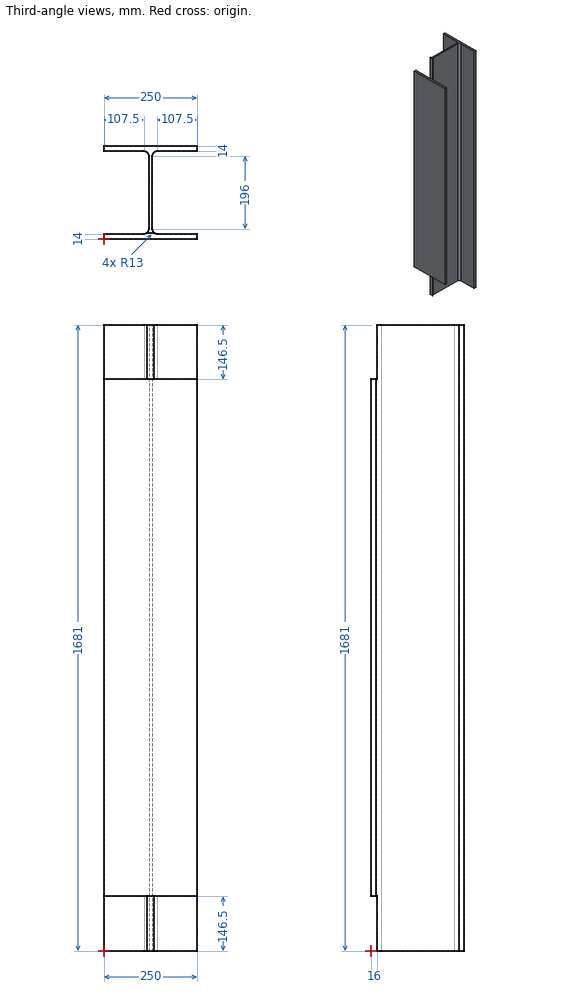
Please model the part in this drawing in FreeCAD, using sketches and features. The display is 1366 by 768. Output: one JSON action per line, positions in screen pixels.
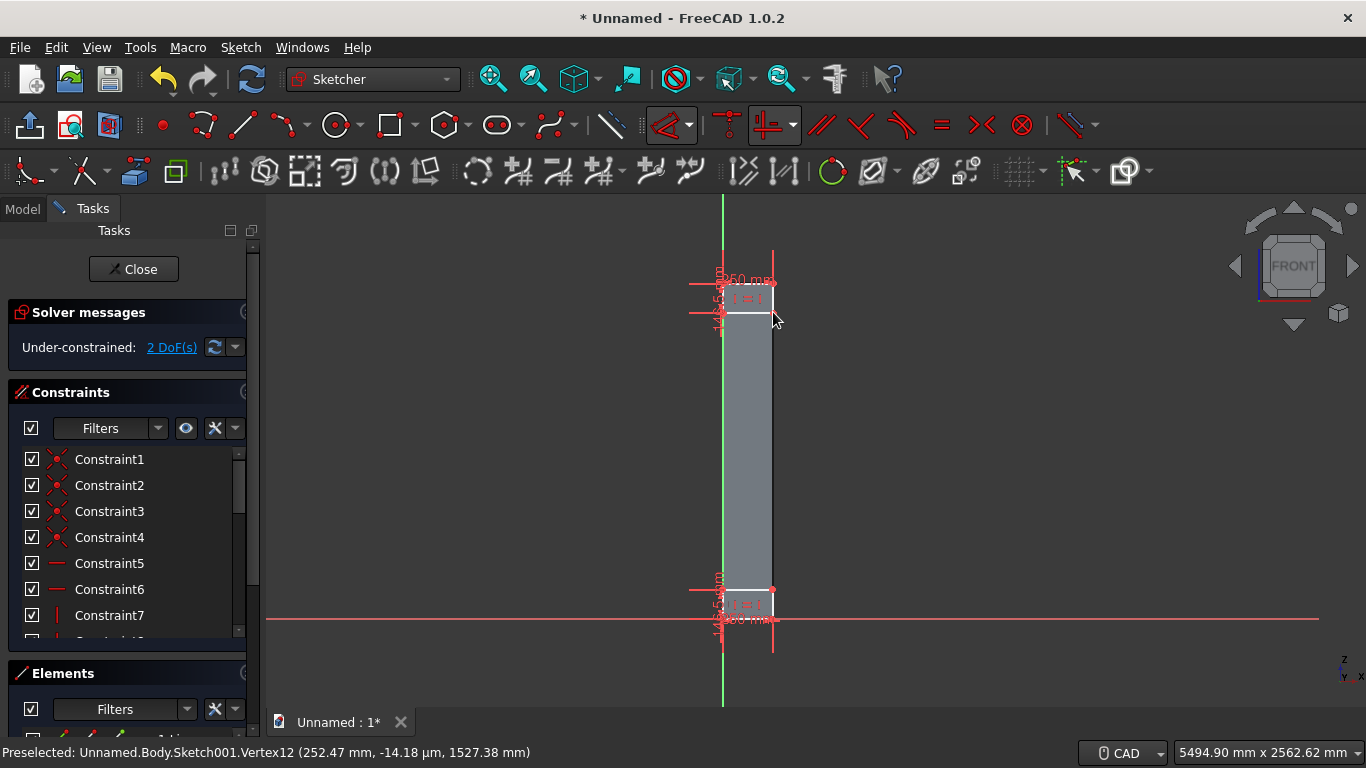
{"action": "left_click", "coordinate": [723, 284]}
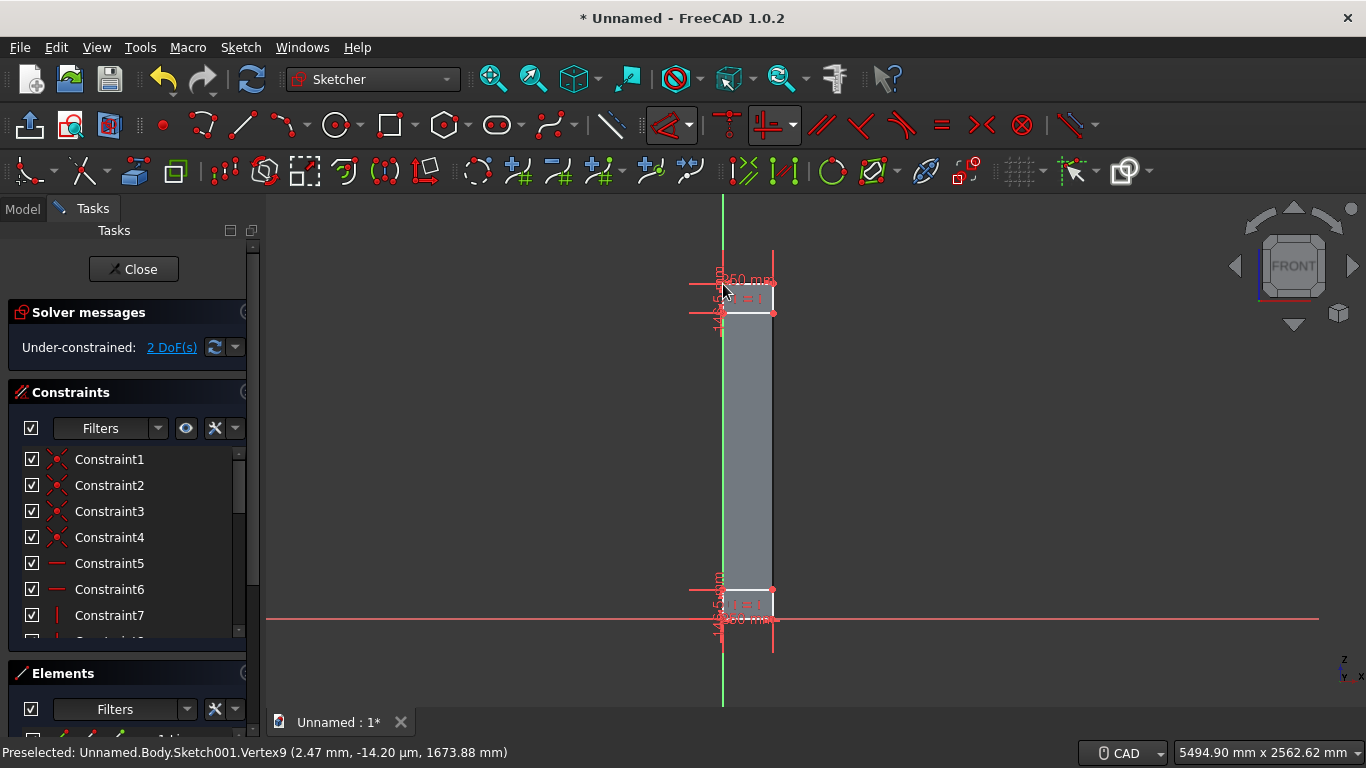
{"action": "left_click", "coordinate": [723, 548]}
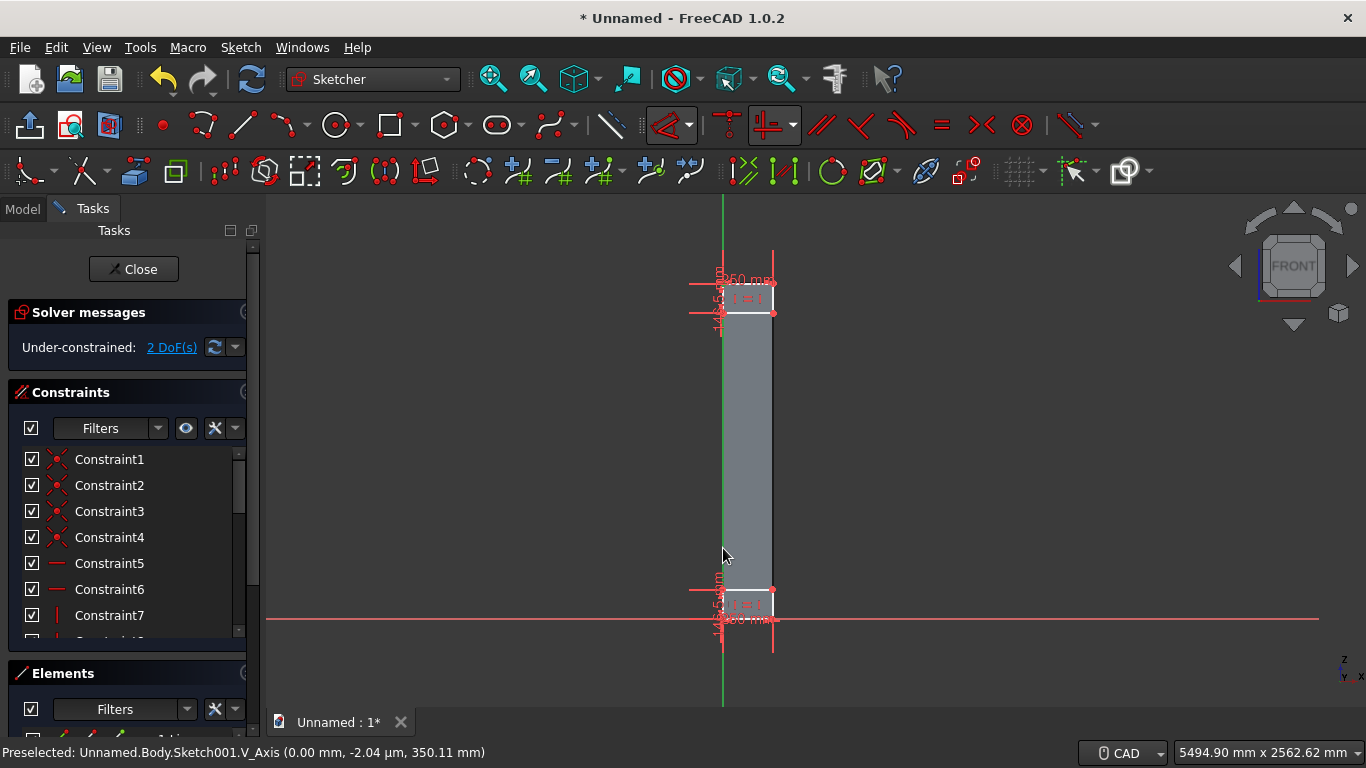
{"action": "left_click", "coordinate": [728, 126]}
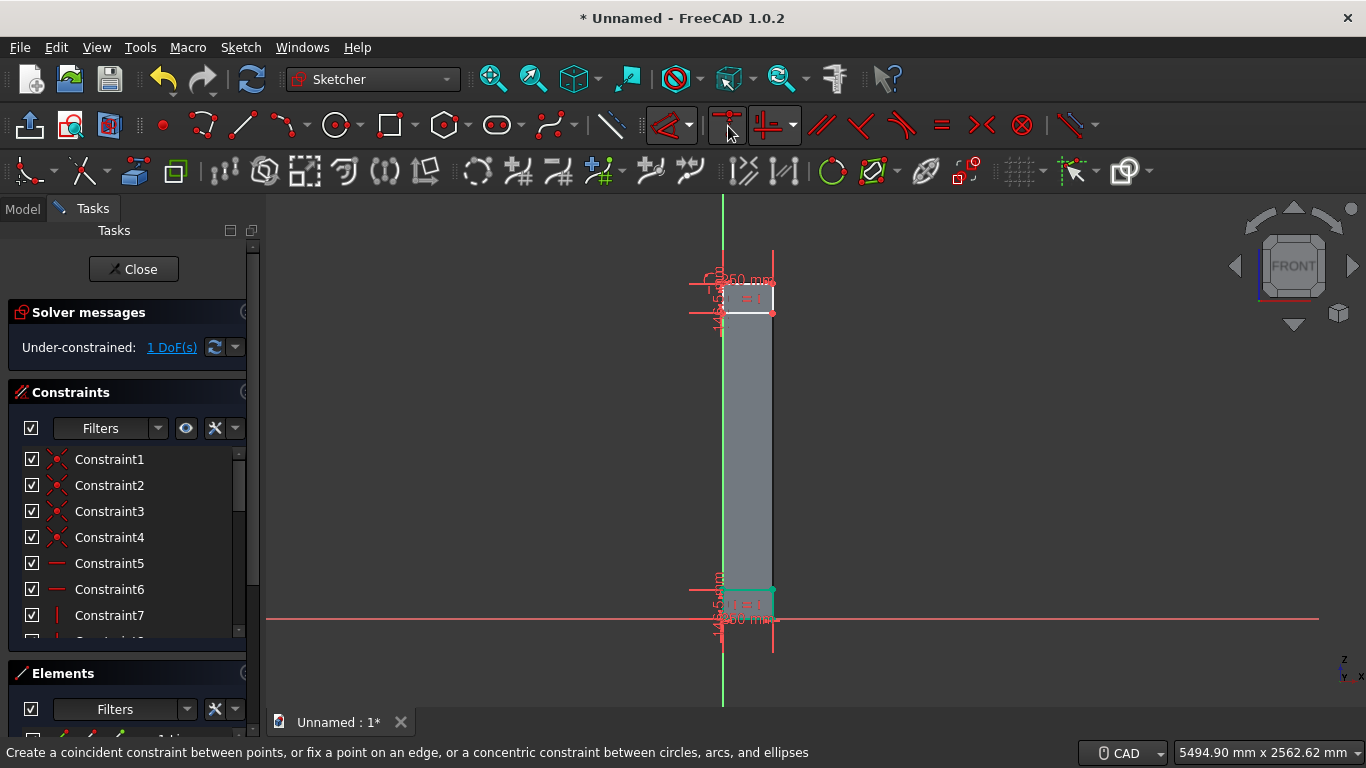
{"action": "left_click", "coordinate": [723, 284]}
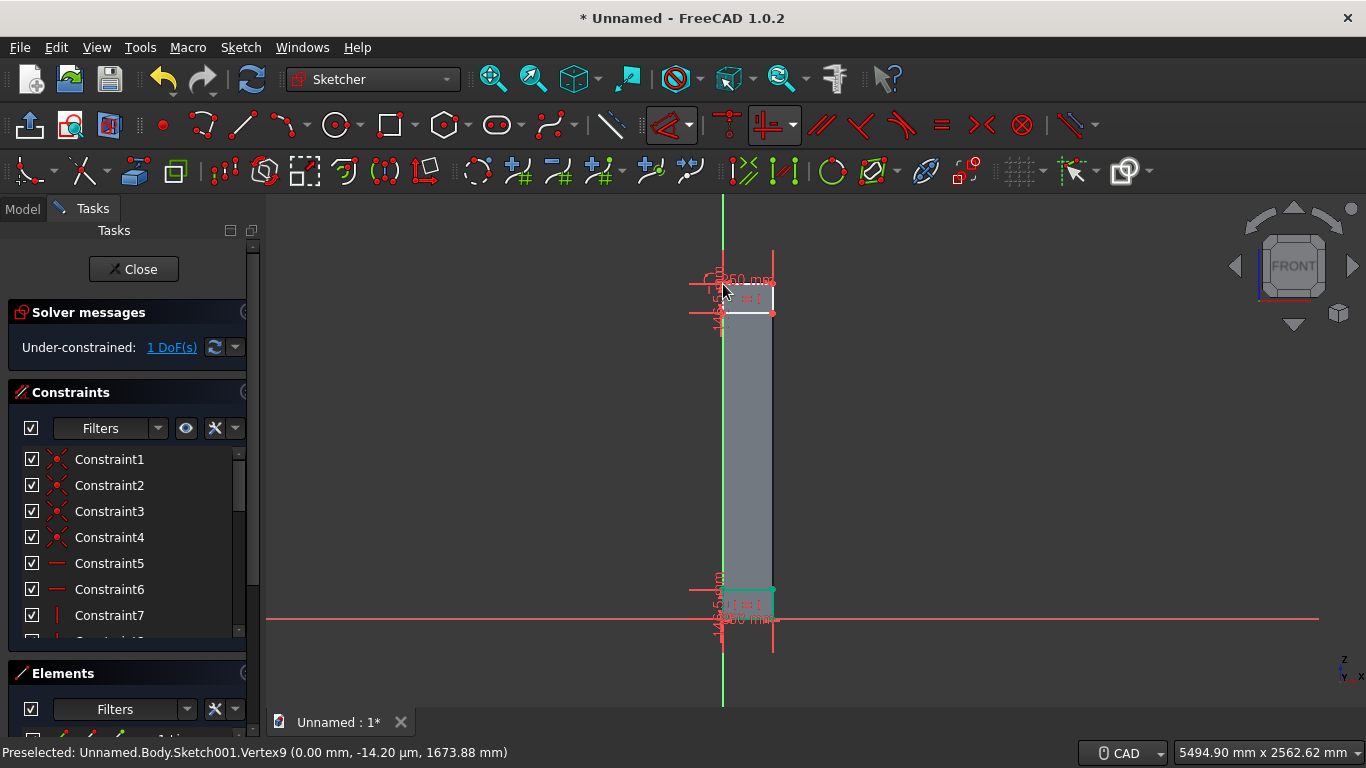
{"action": "key", "text": "i"}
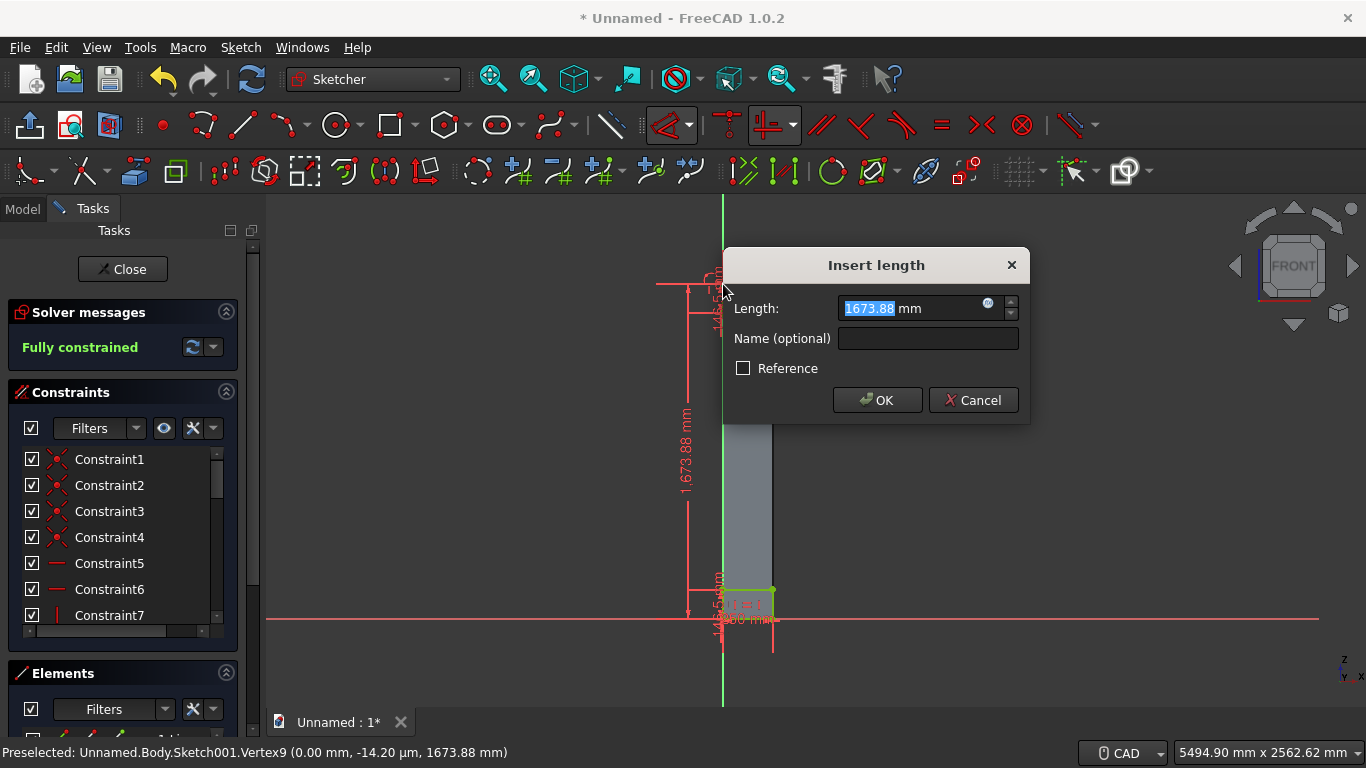
{"action": "type", "text": "1681"}
{"action": "key", "text": "Return"}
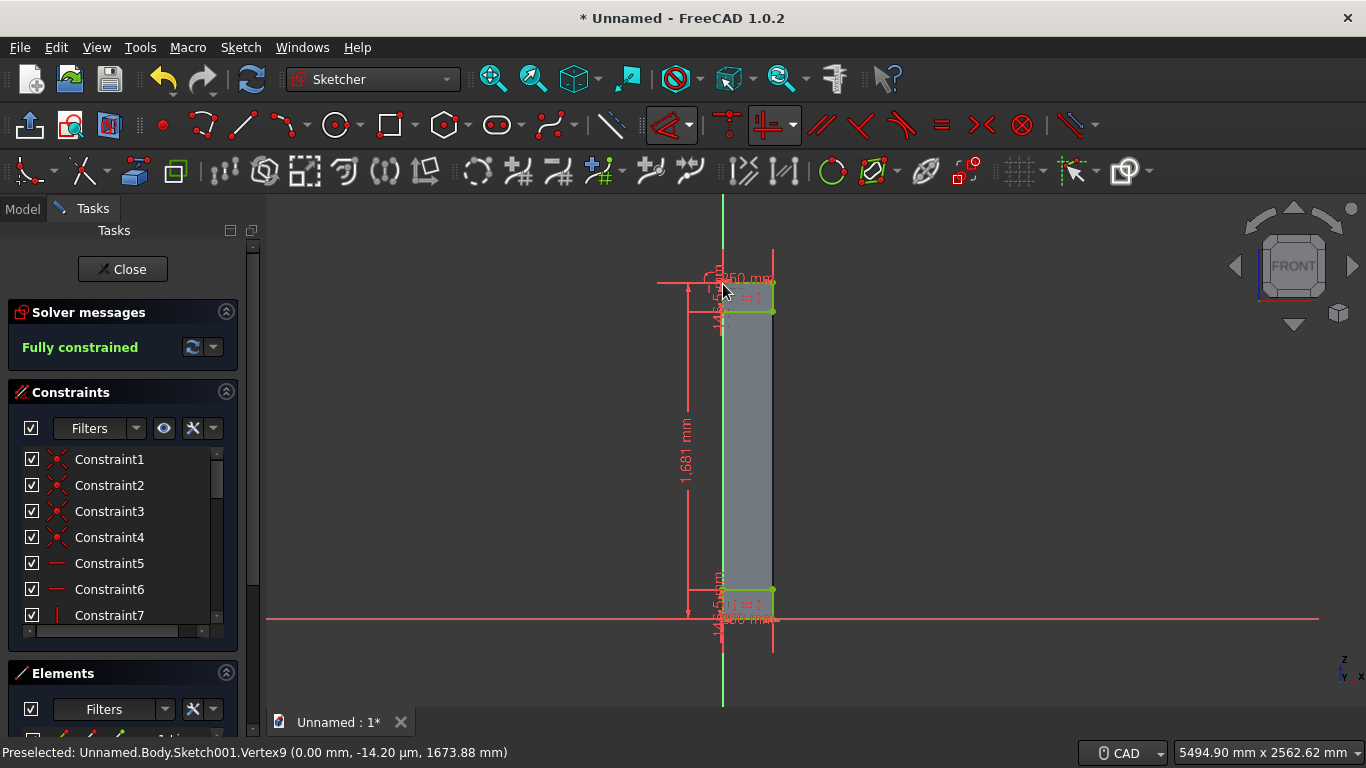
{"action": "left_click", "coordinate": [123, 269]}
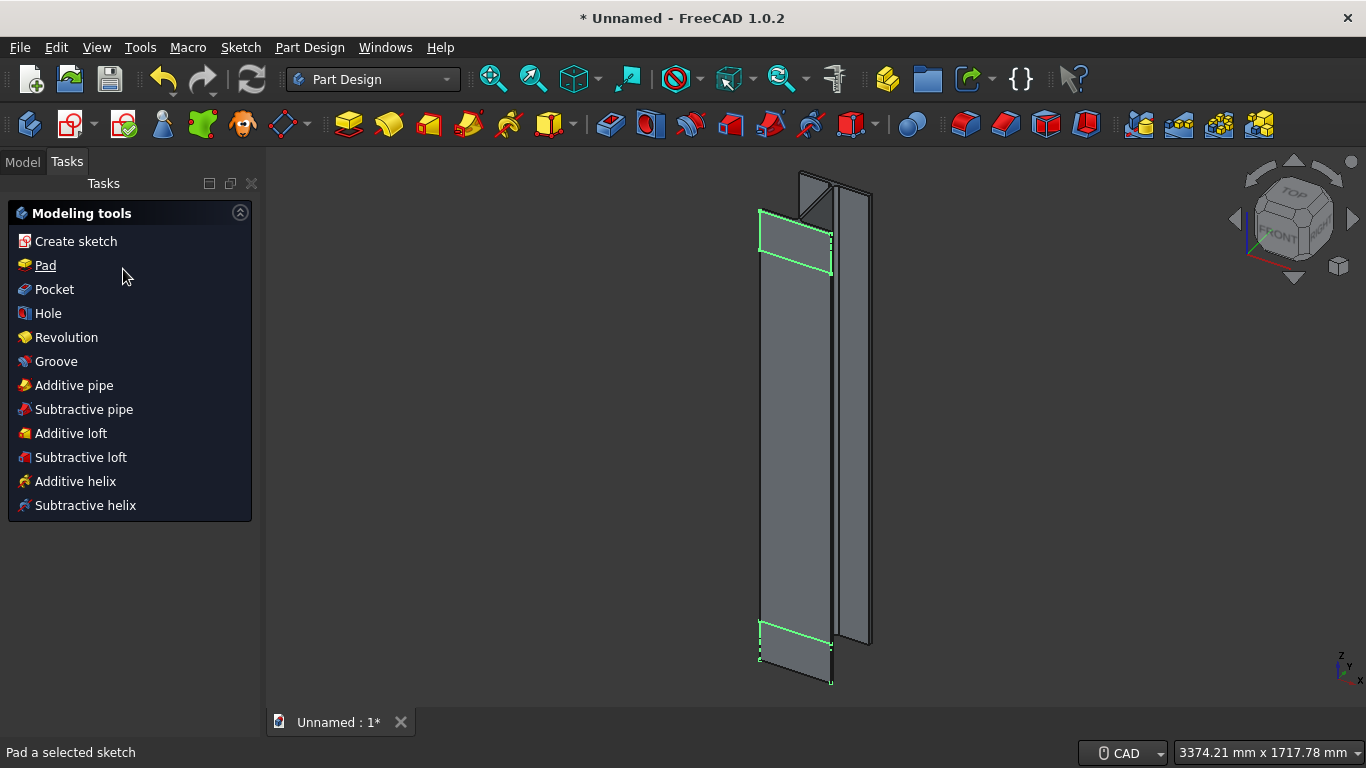
{"action": "left_click", "coordinate": [612, 124]}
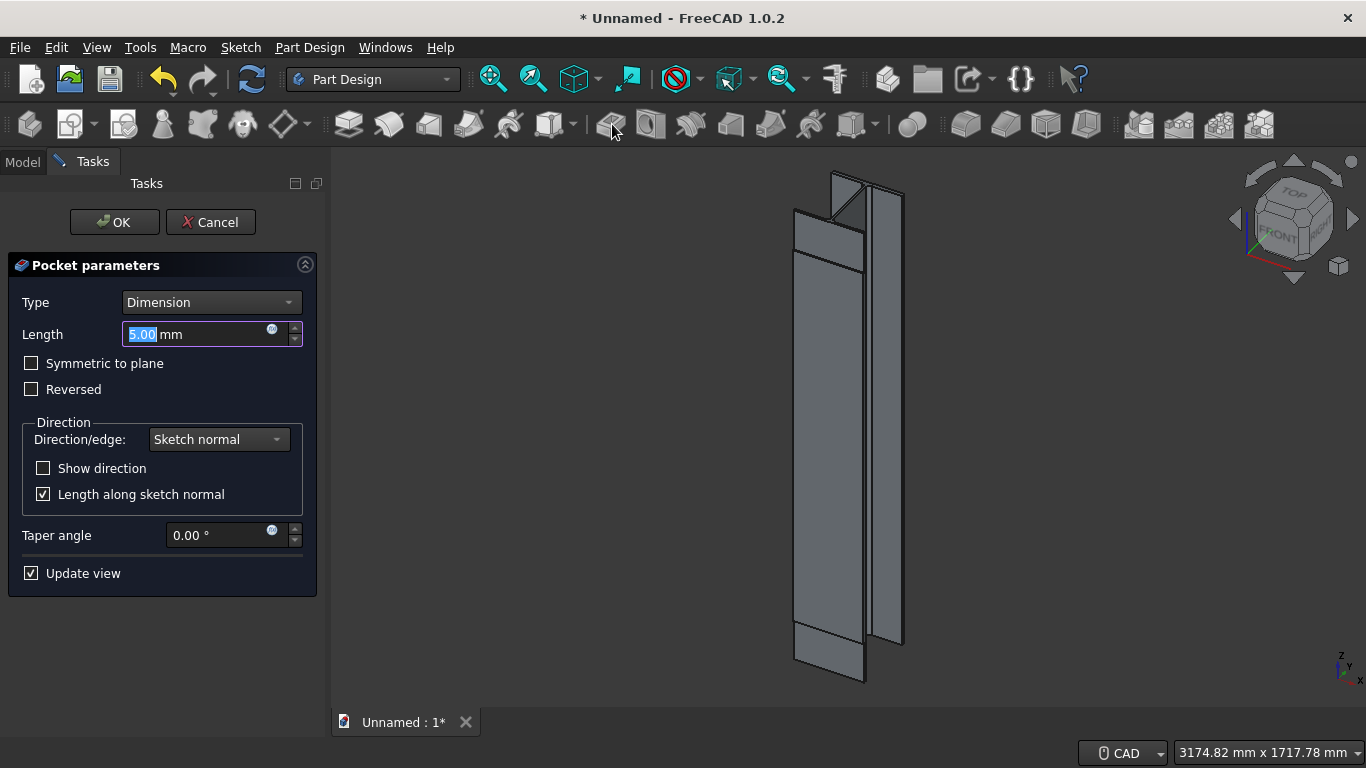
{"action": "type", "text": "16"}
{"action": "key", "text": "Tab"}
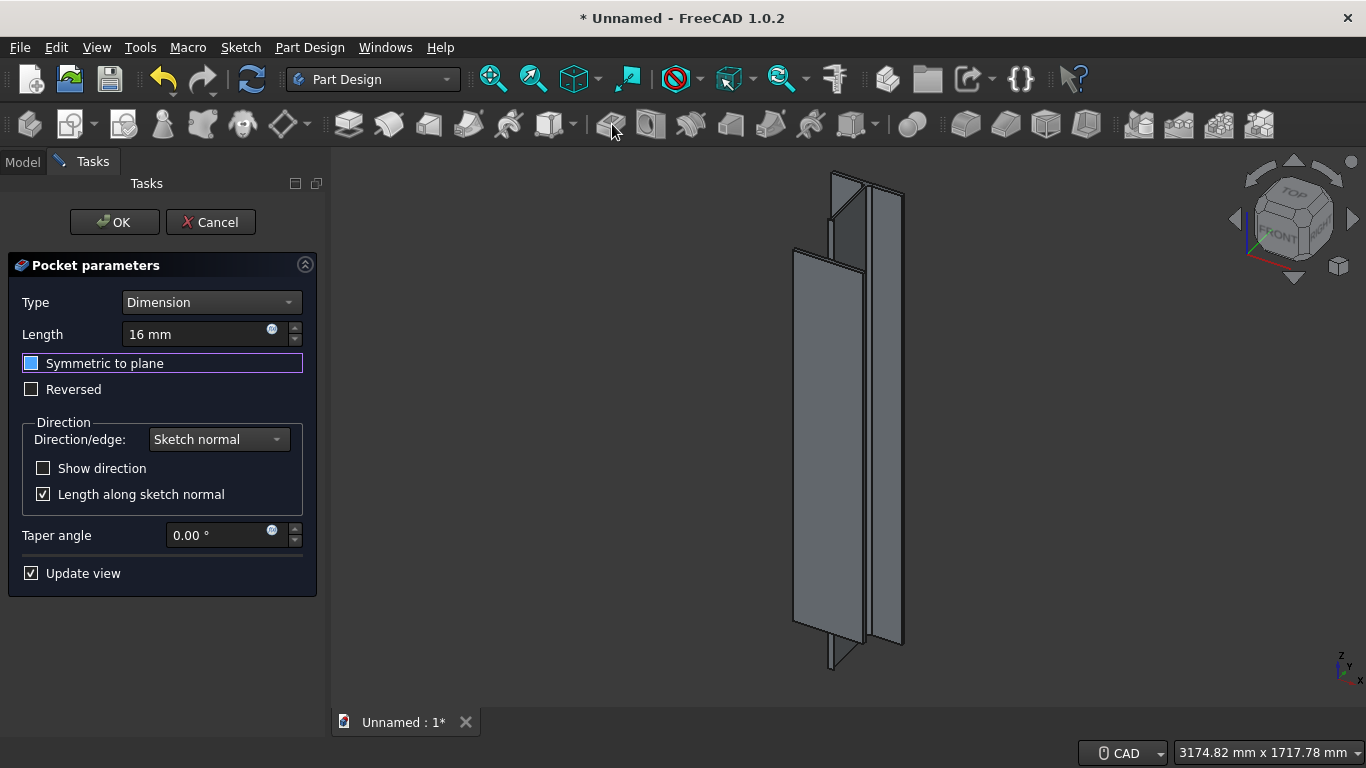
{"action": "left_click", "coordinate": [115, 222]}